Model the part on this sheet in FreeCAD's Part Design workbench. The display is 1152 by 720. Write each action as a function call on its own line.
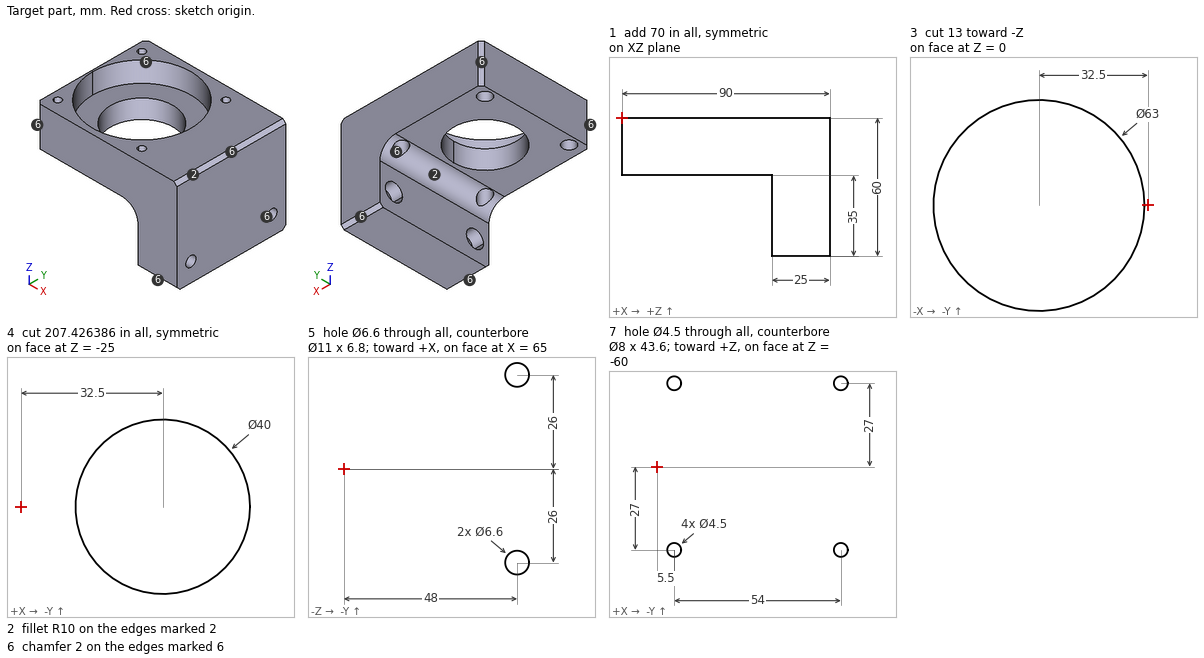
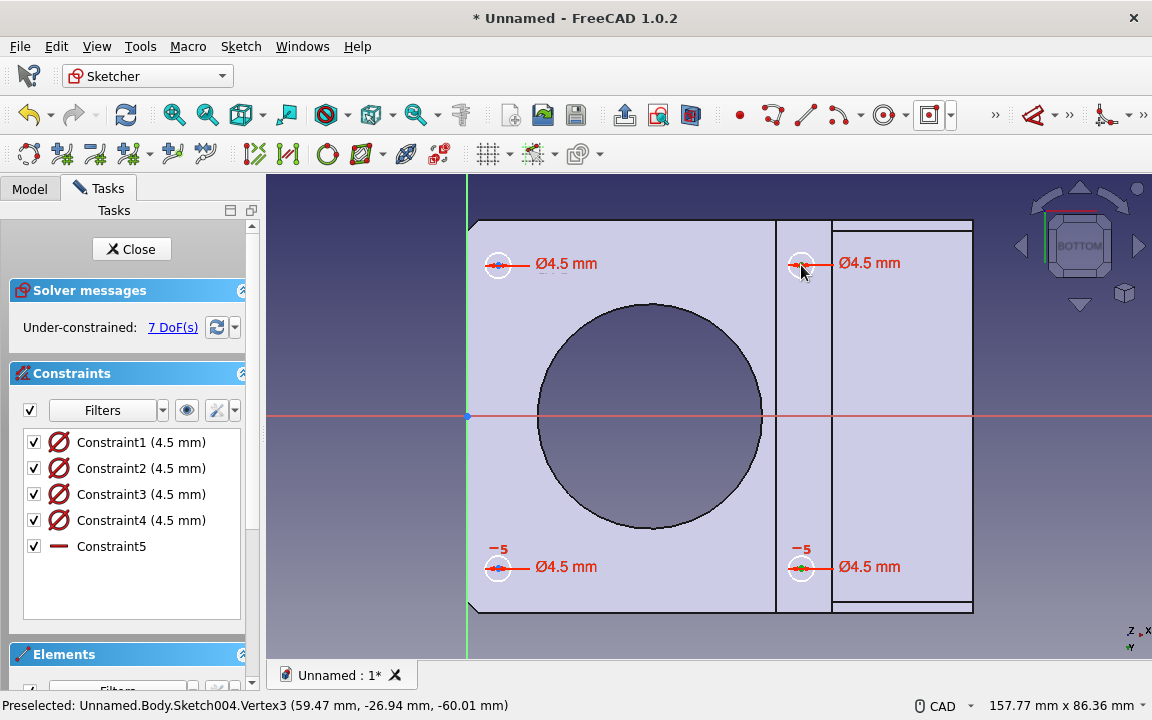
key(v)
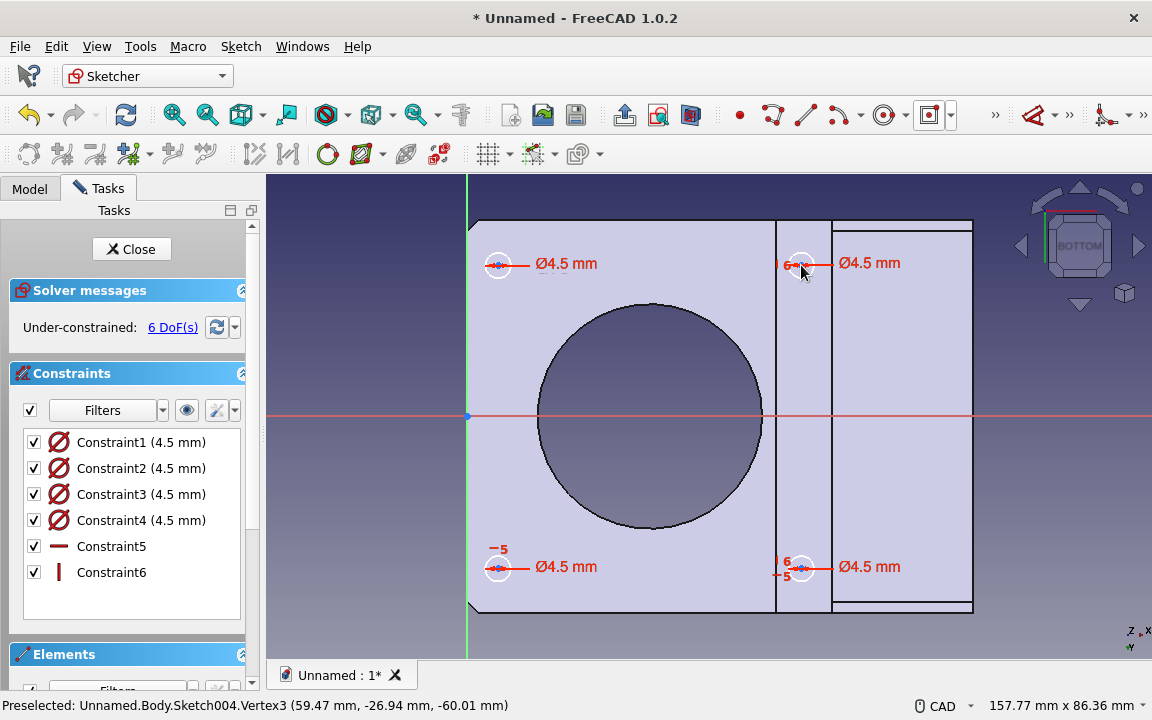
click(498, 569)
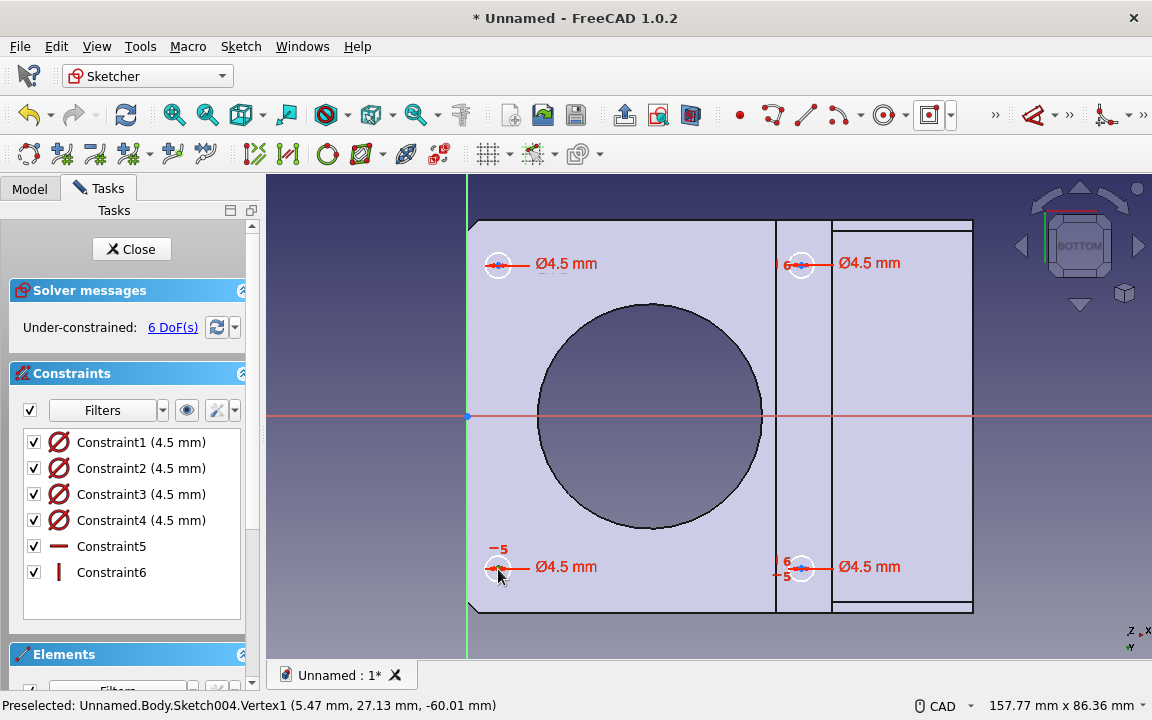
click(498, 266)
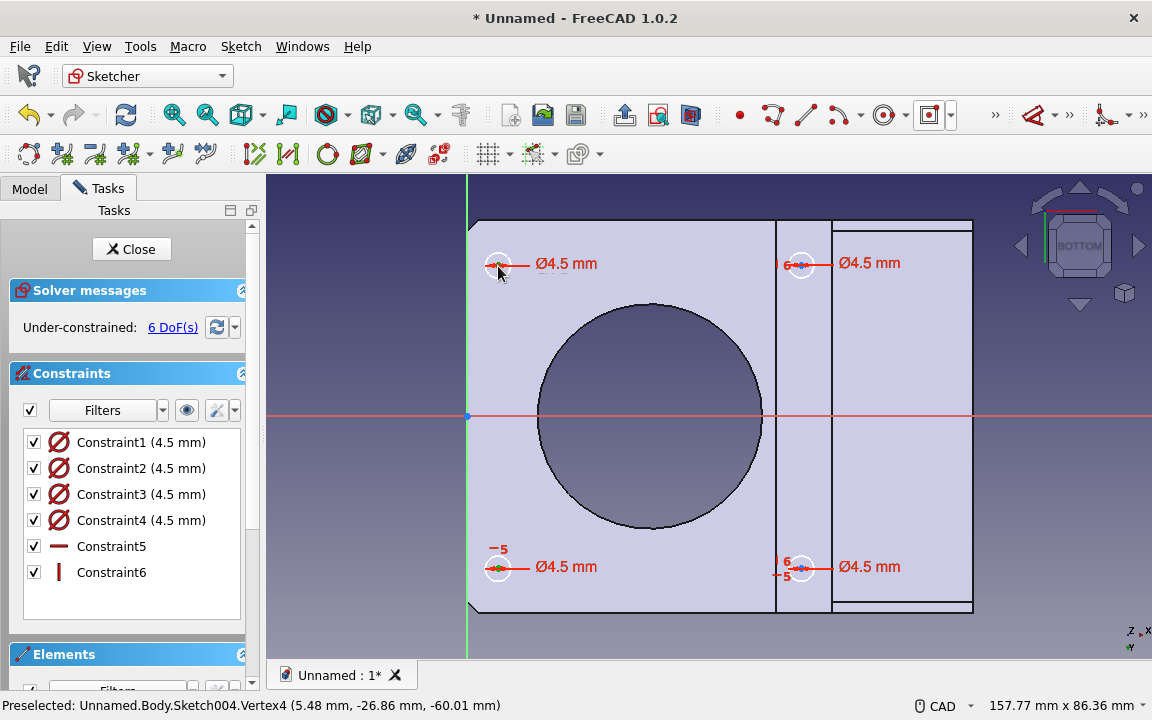
key(v)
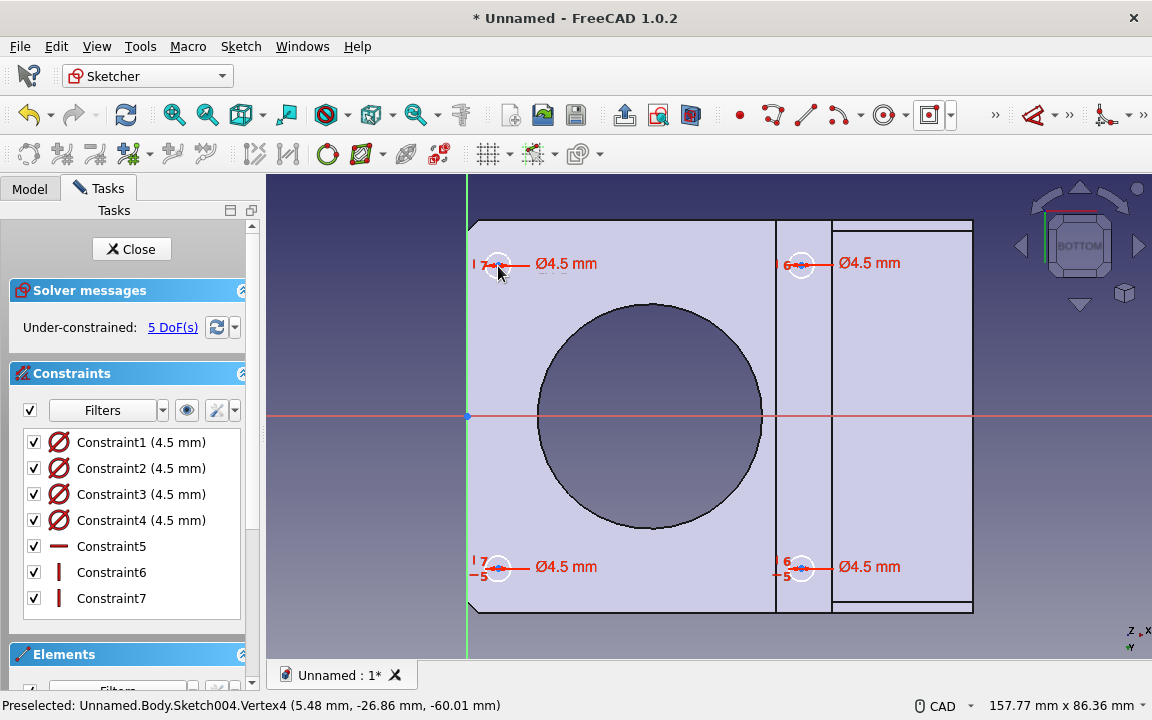
click(801, 265)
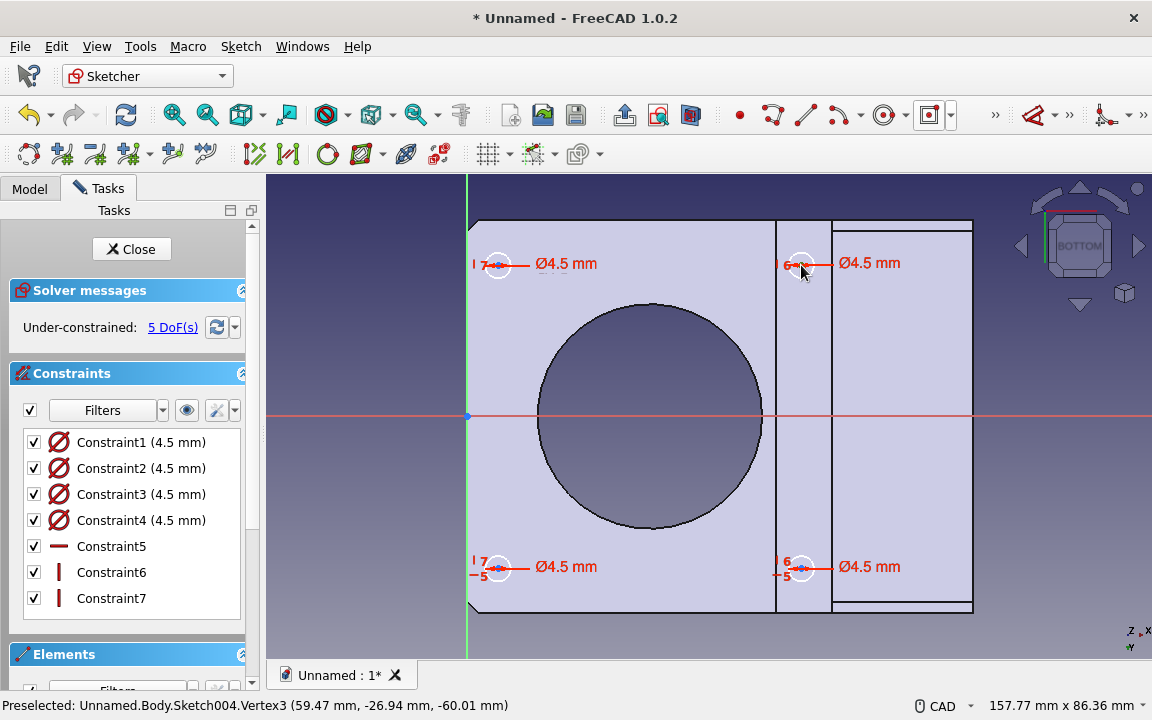
click(498, 266)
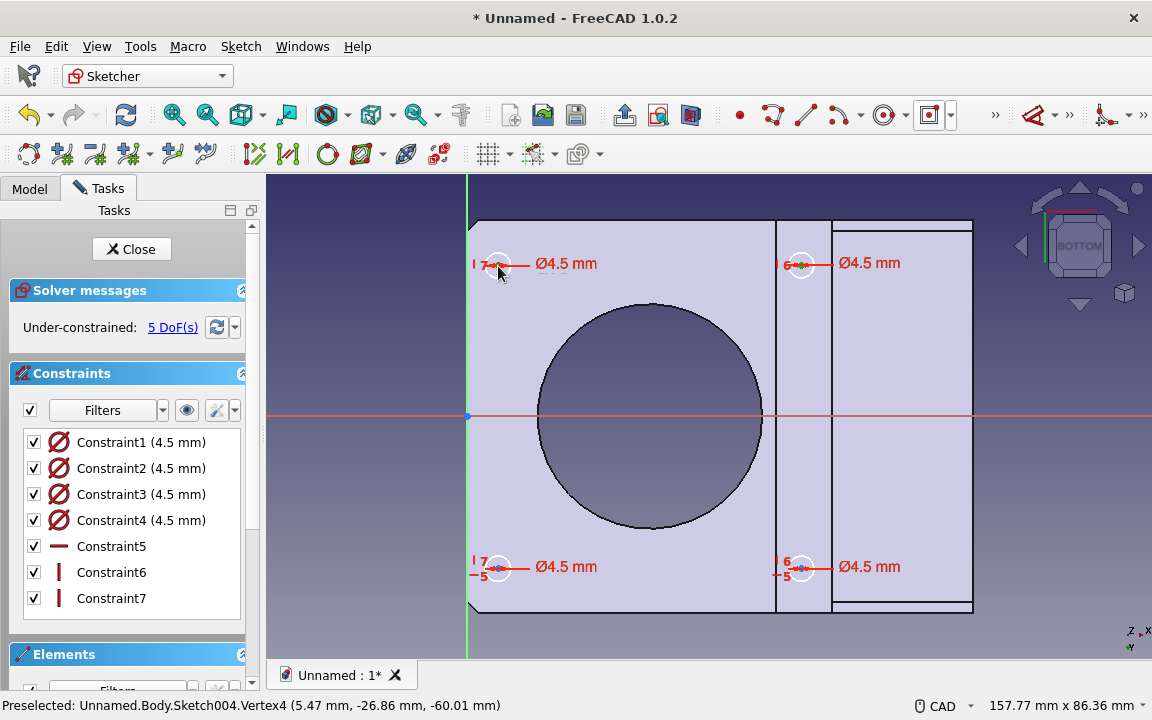
key(h)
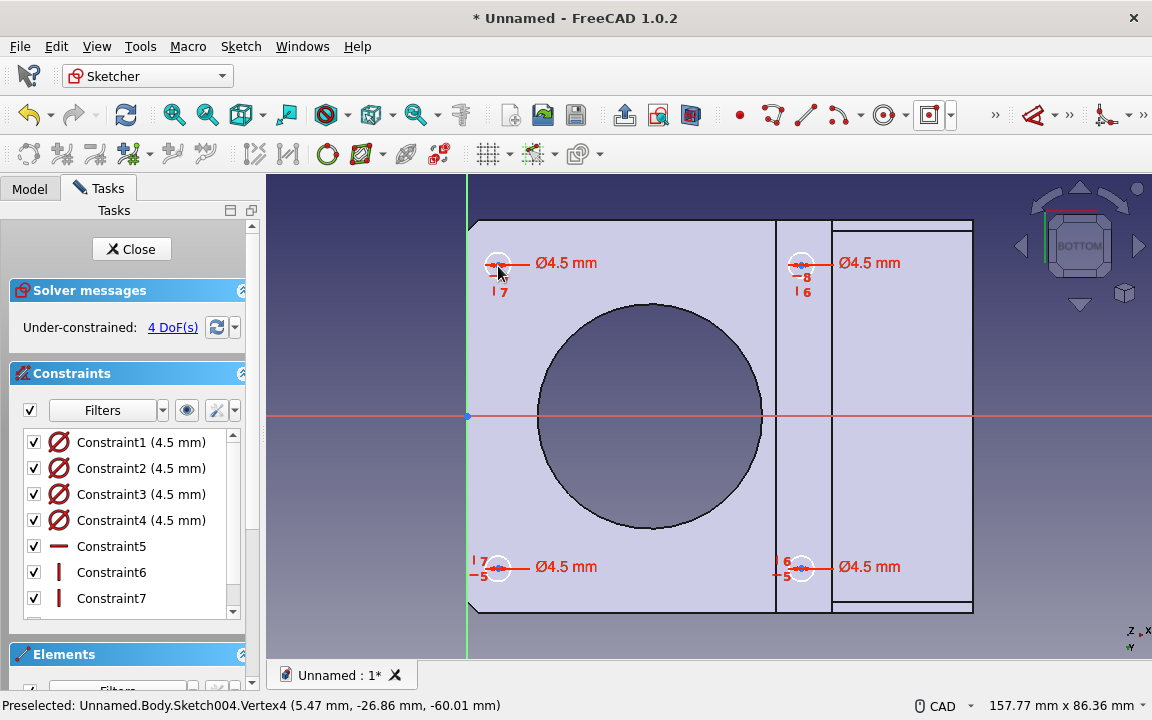
click(1032, 116)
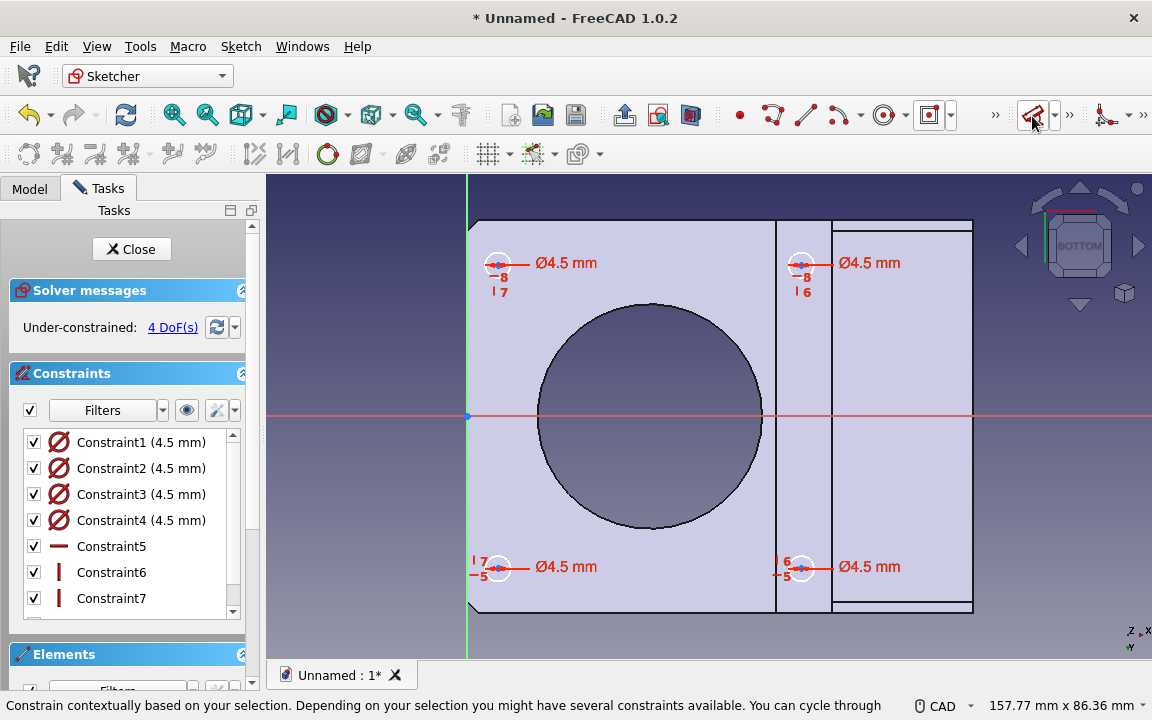
click(498, 569)
click(433, 493)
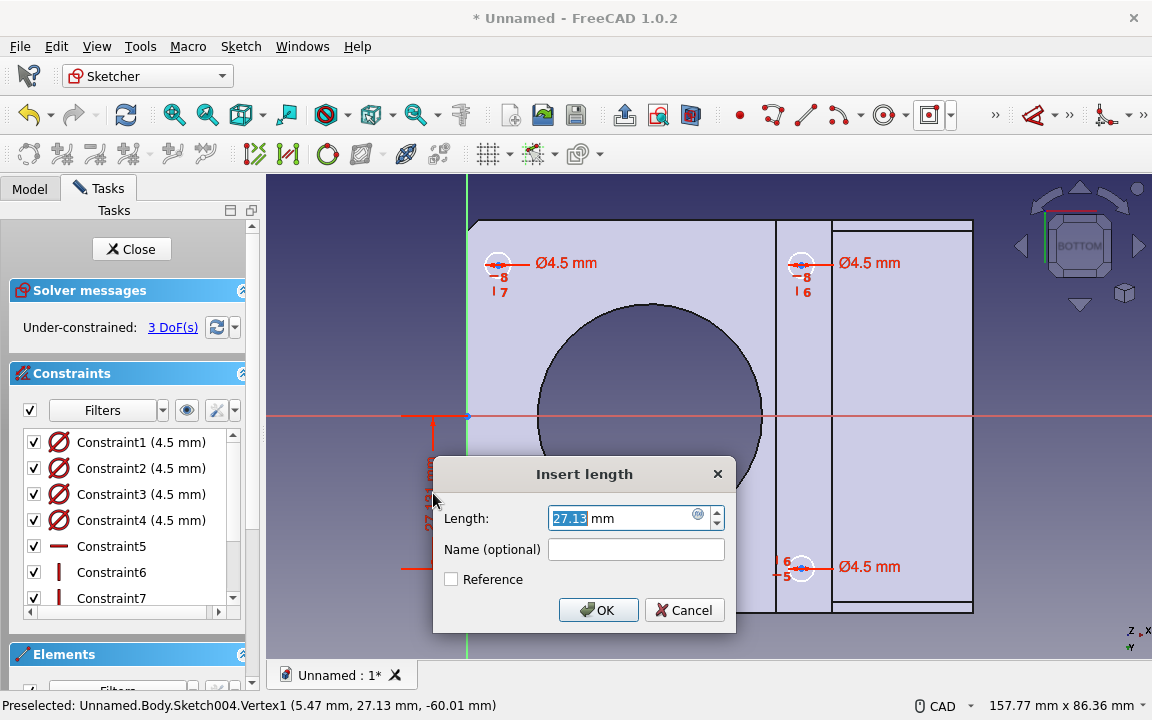
text(27)
key(Return)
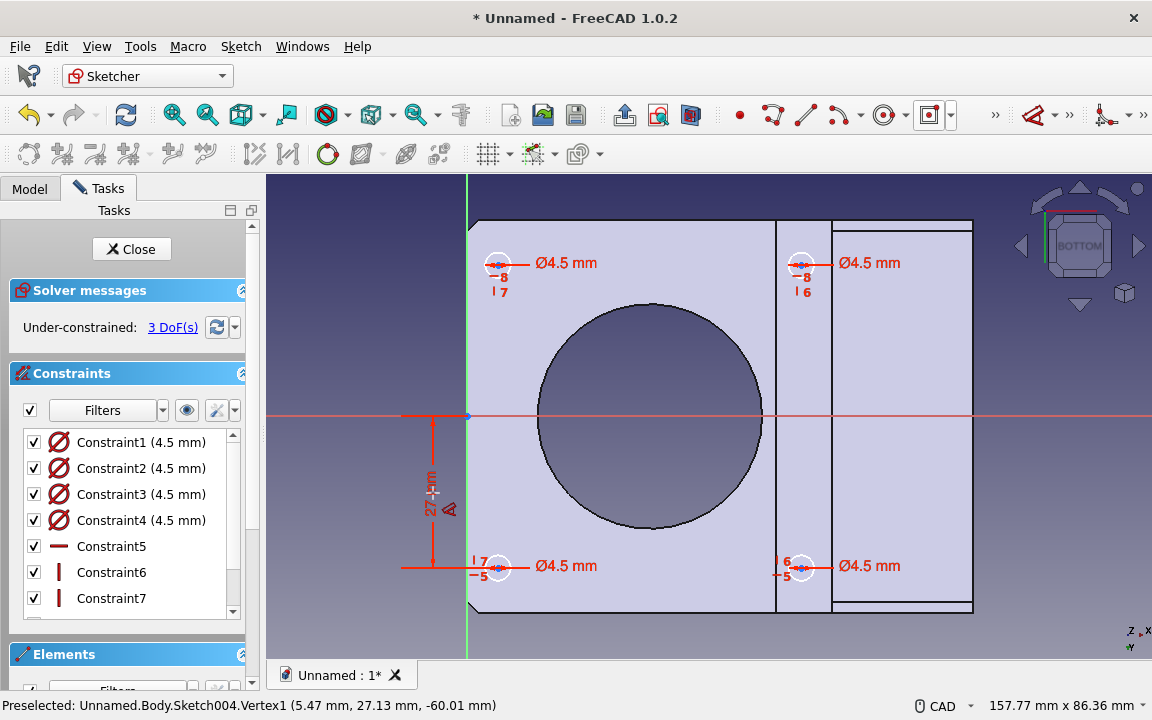
click(801, 265)
click(433, 341)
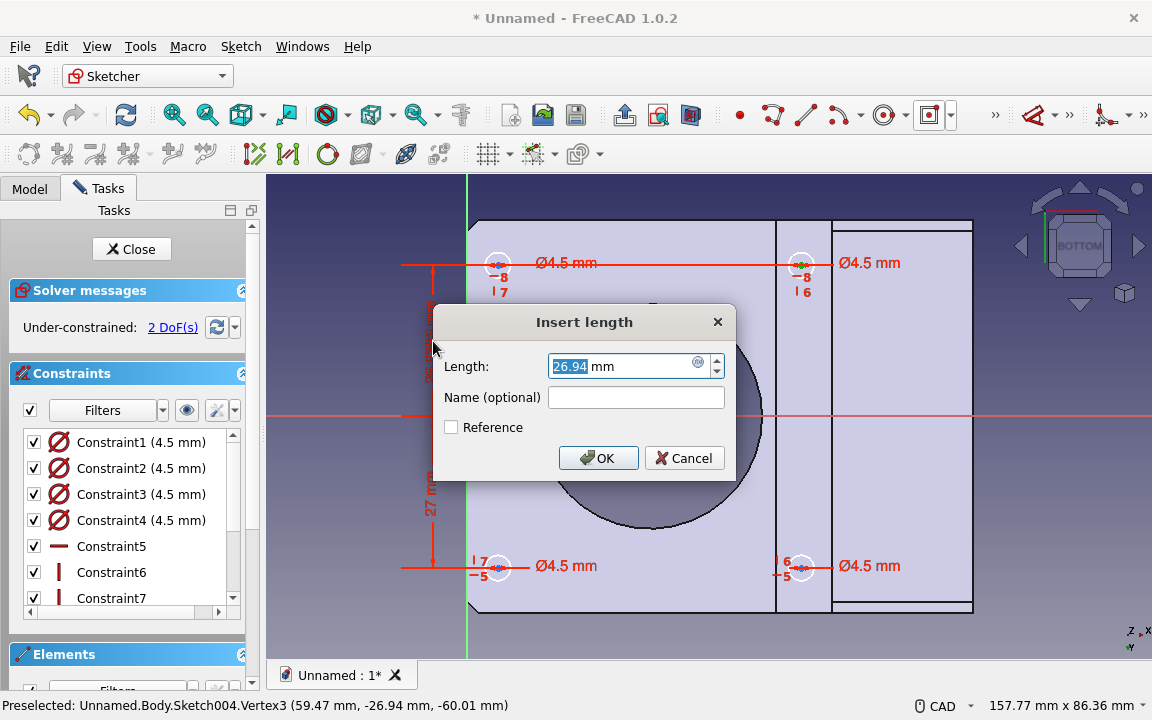
text(27)
key(Return)